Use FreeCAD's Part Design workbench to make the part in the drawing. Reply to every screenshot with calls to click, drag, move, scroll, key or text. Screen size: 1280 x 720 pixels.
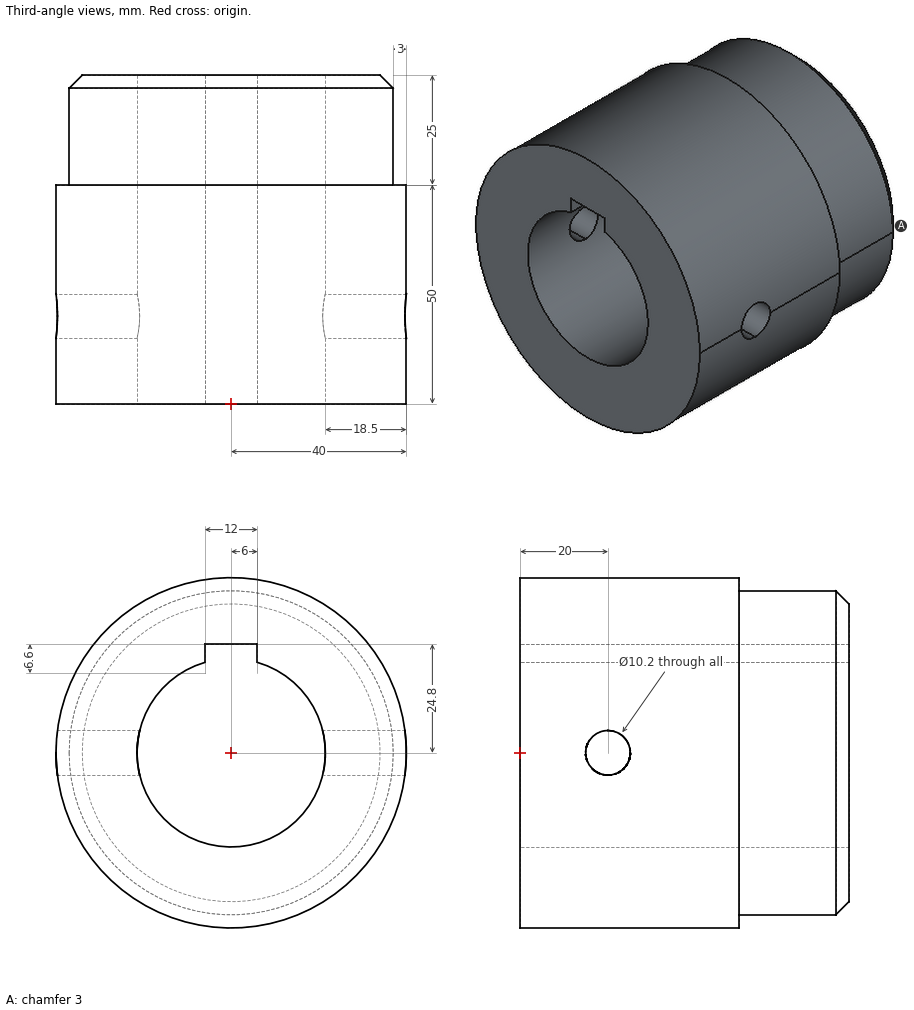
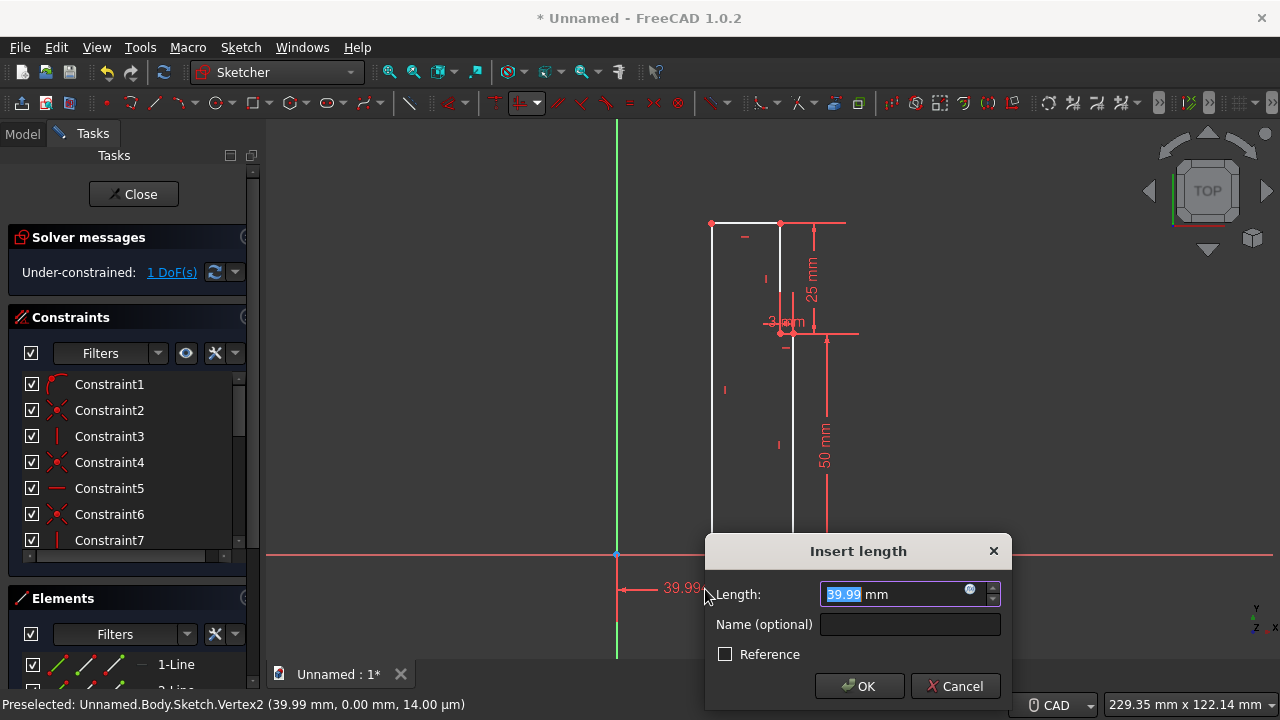
text(40)
key(Return)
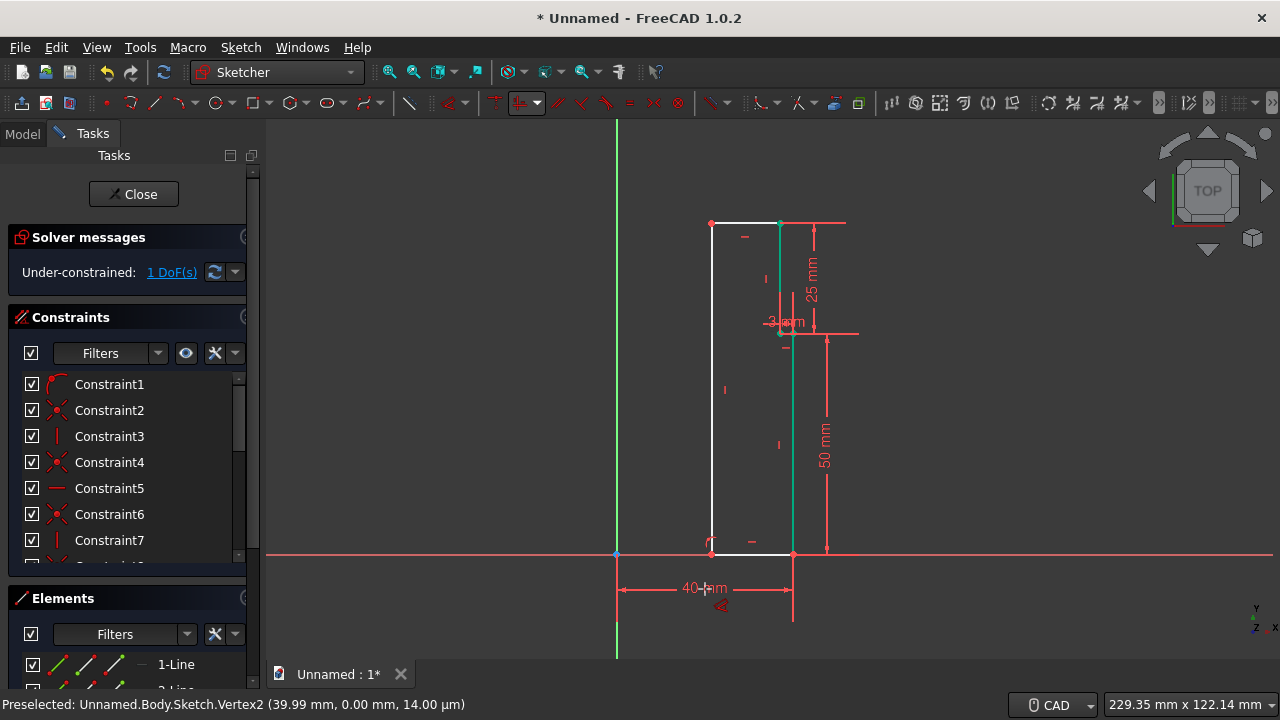
click(736, 555)
click(781, 589)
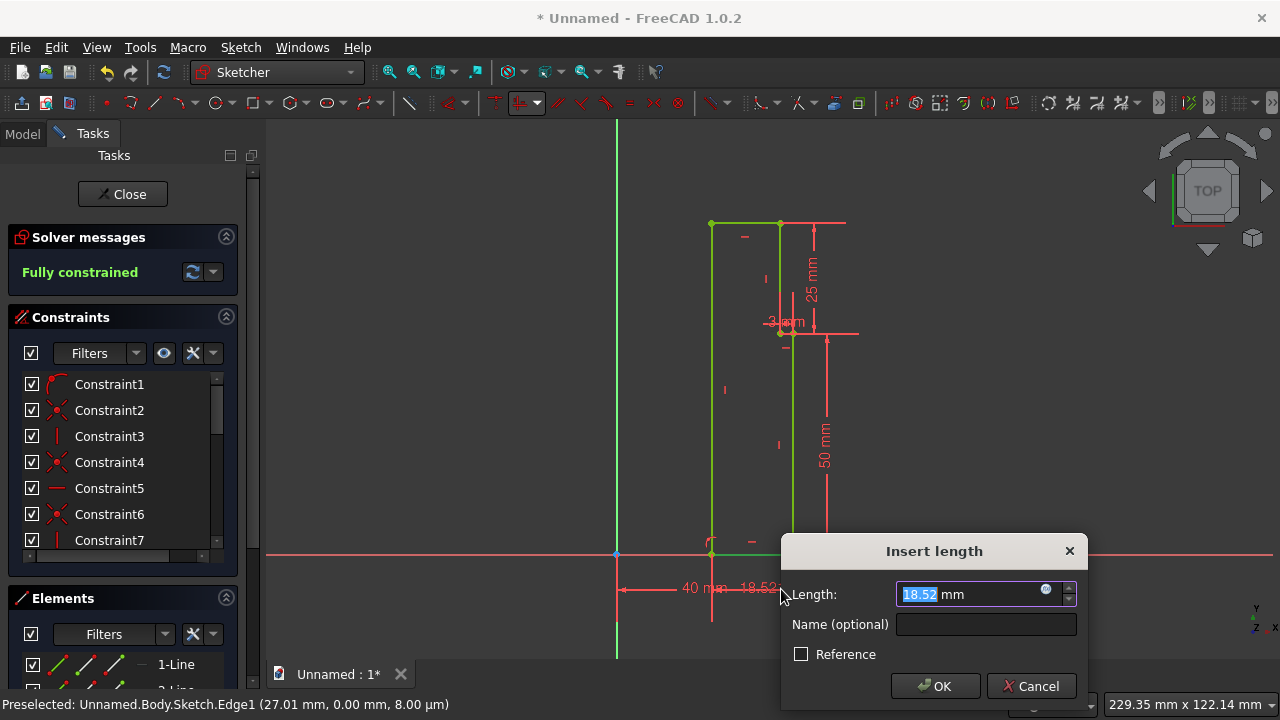
text(18.5)
key(Return)
key(Escape)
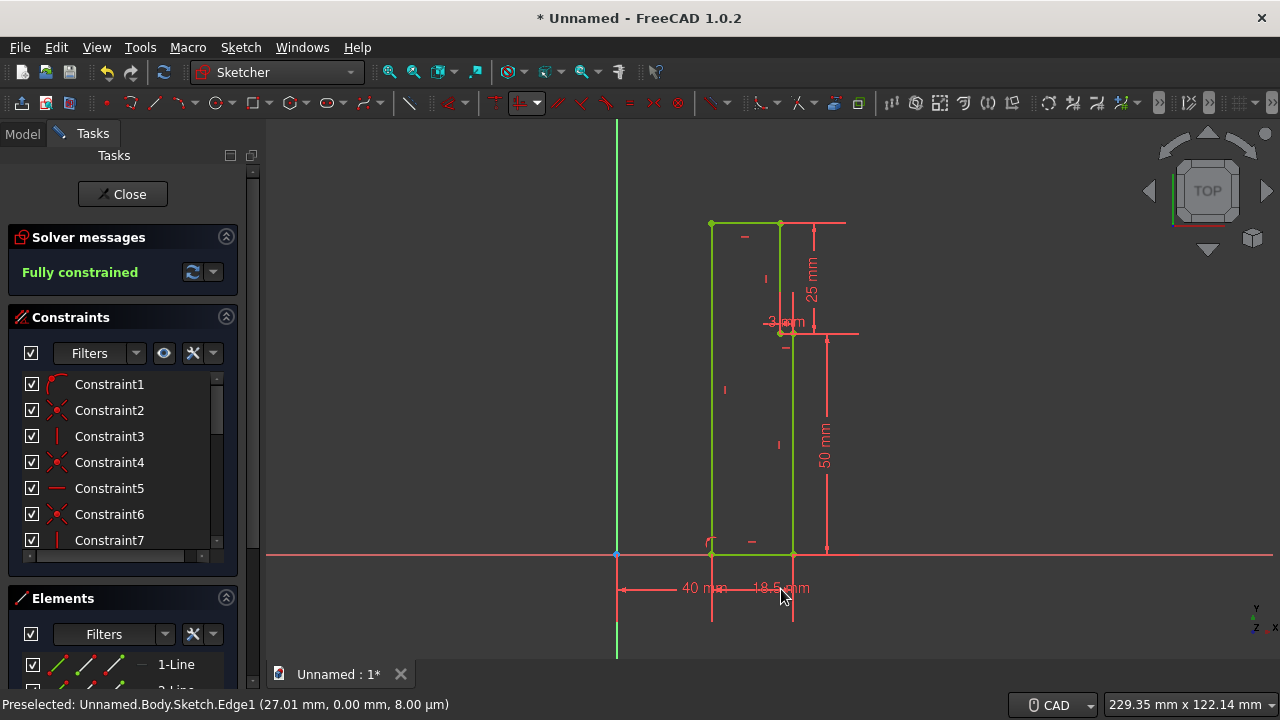
click(123, 194)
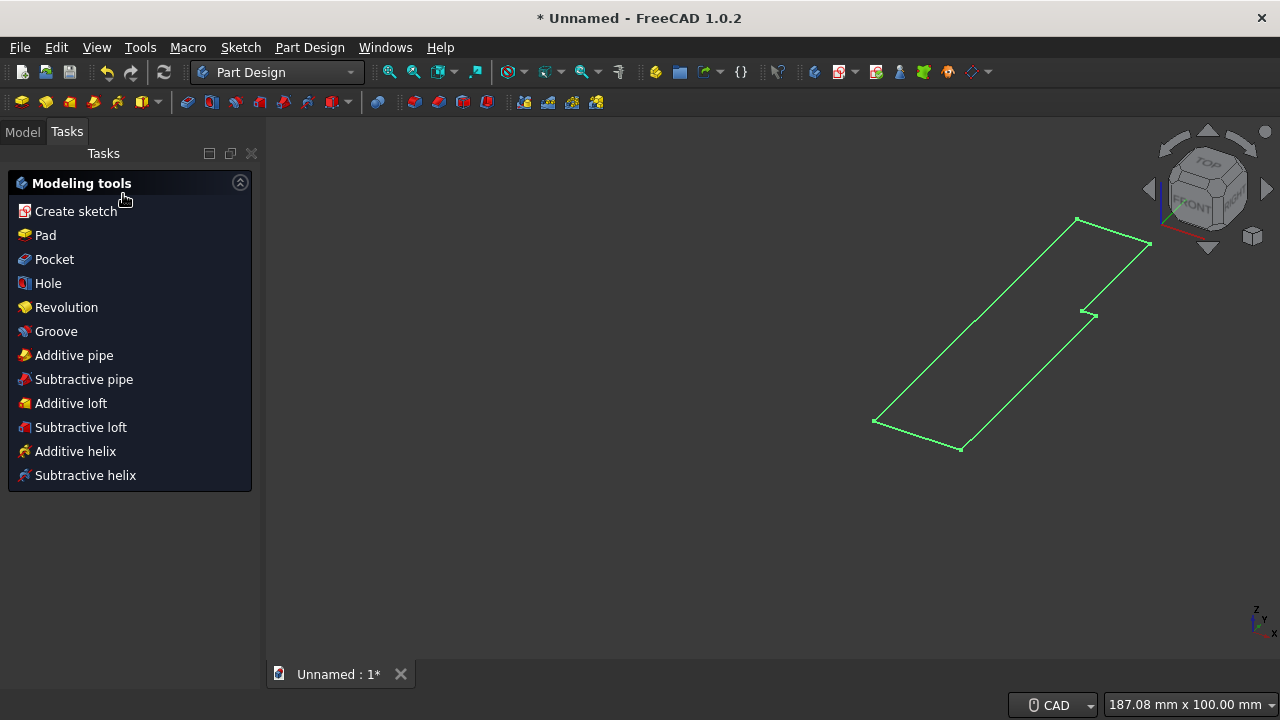
click(46, 102)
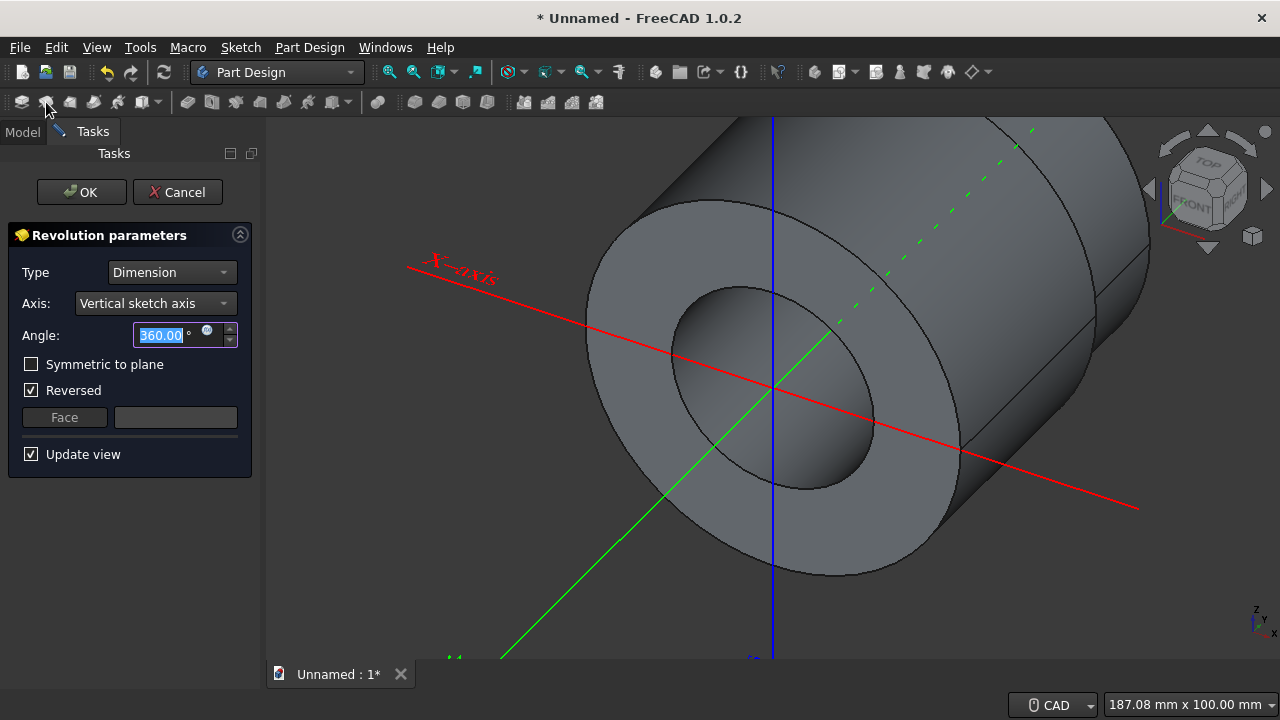
click(82, 192)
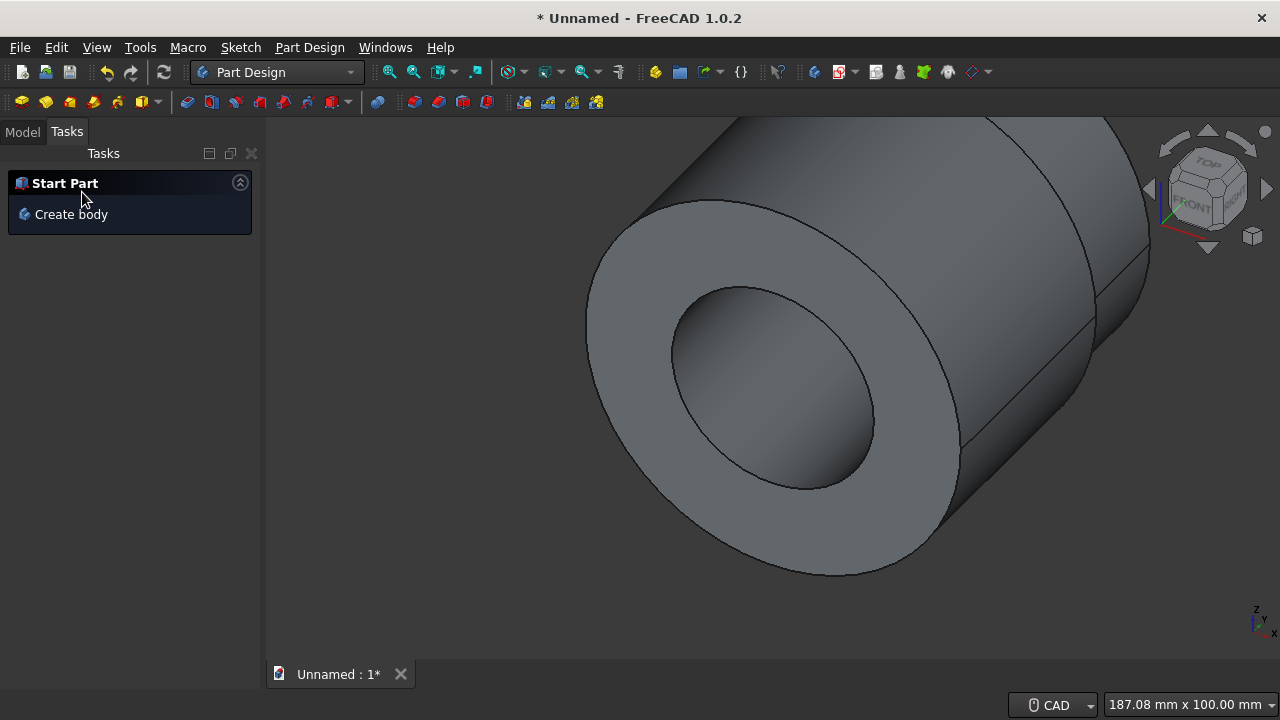
click(390, 72)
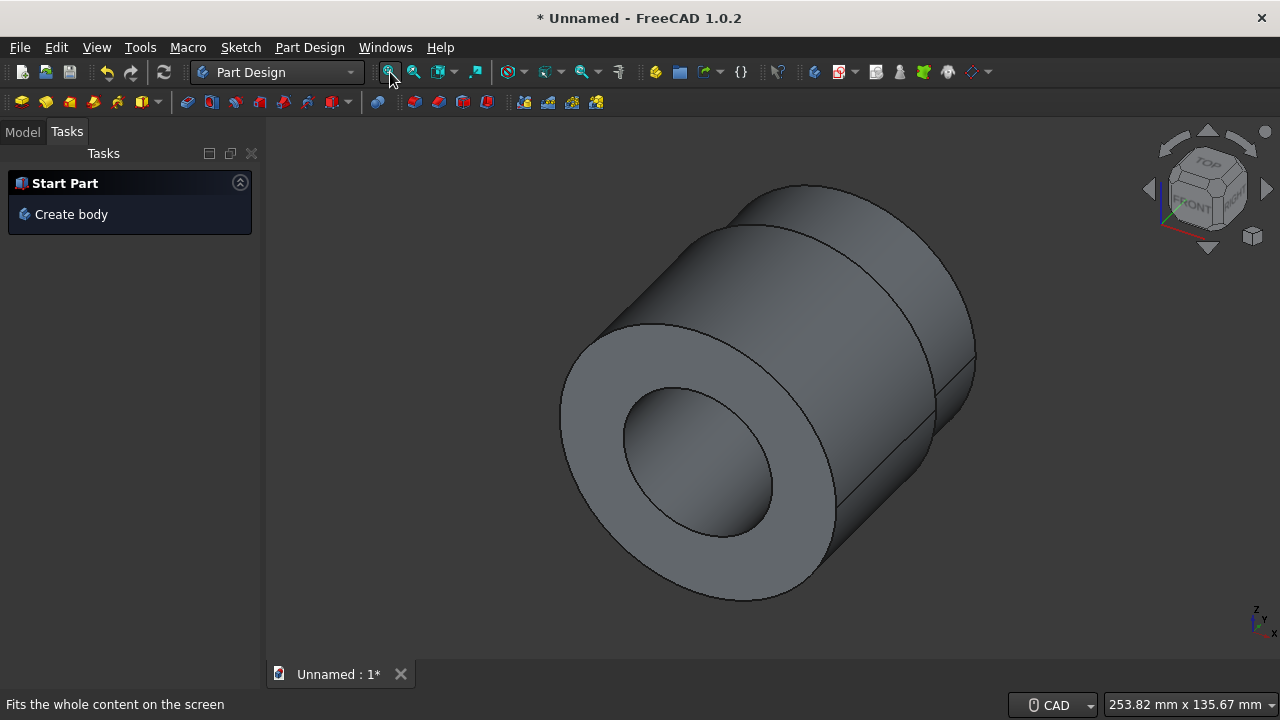
key(0)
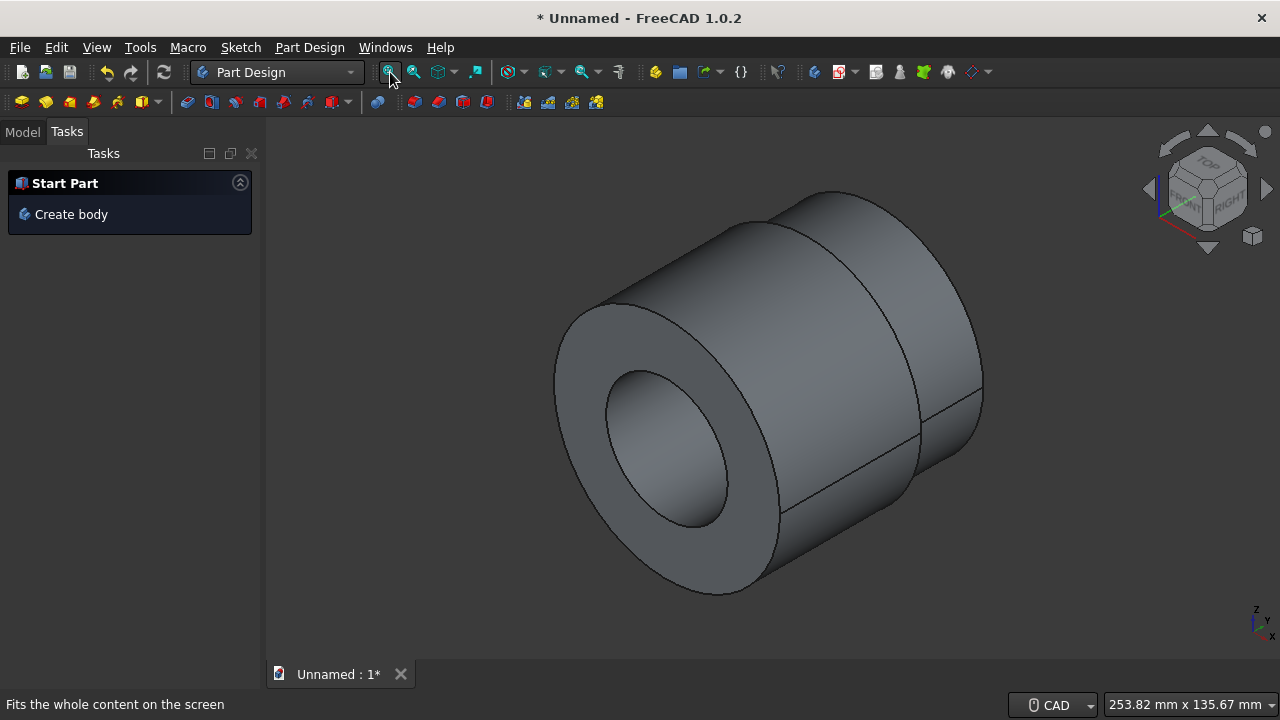
key(2)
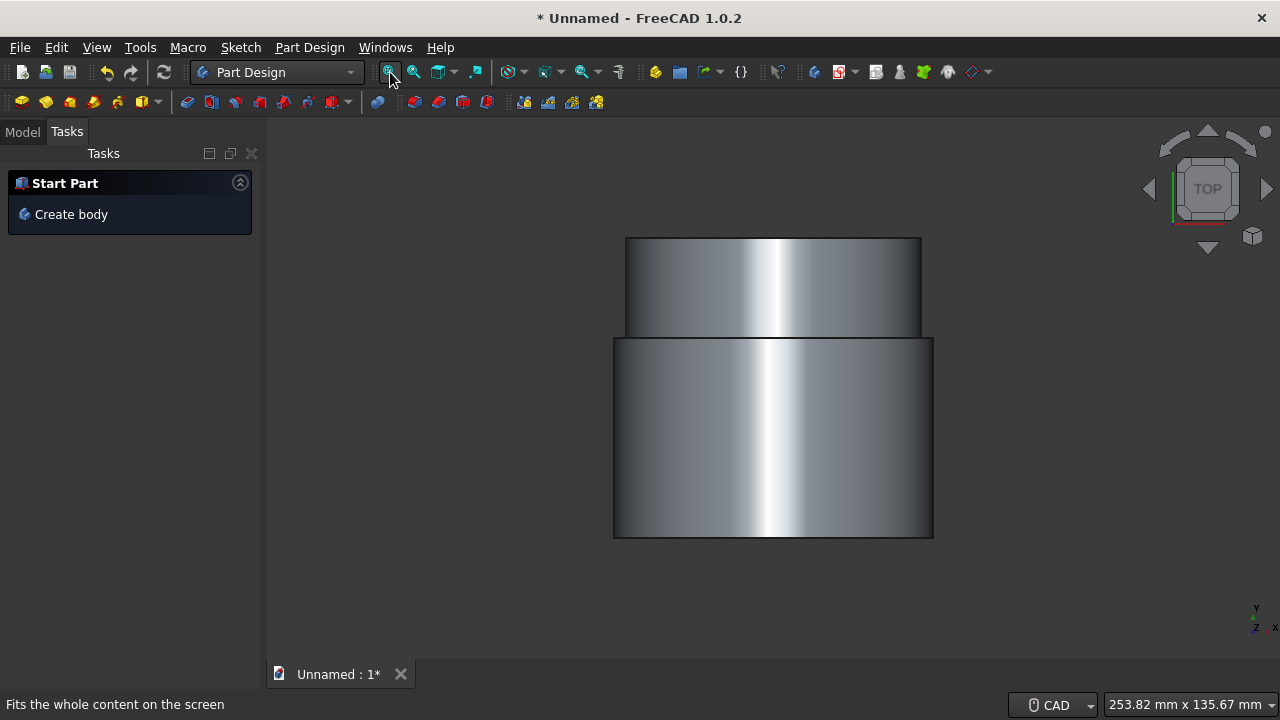
click(653, 237)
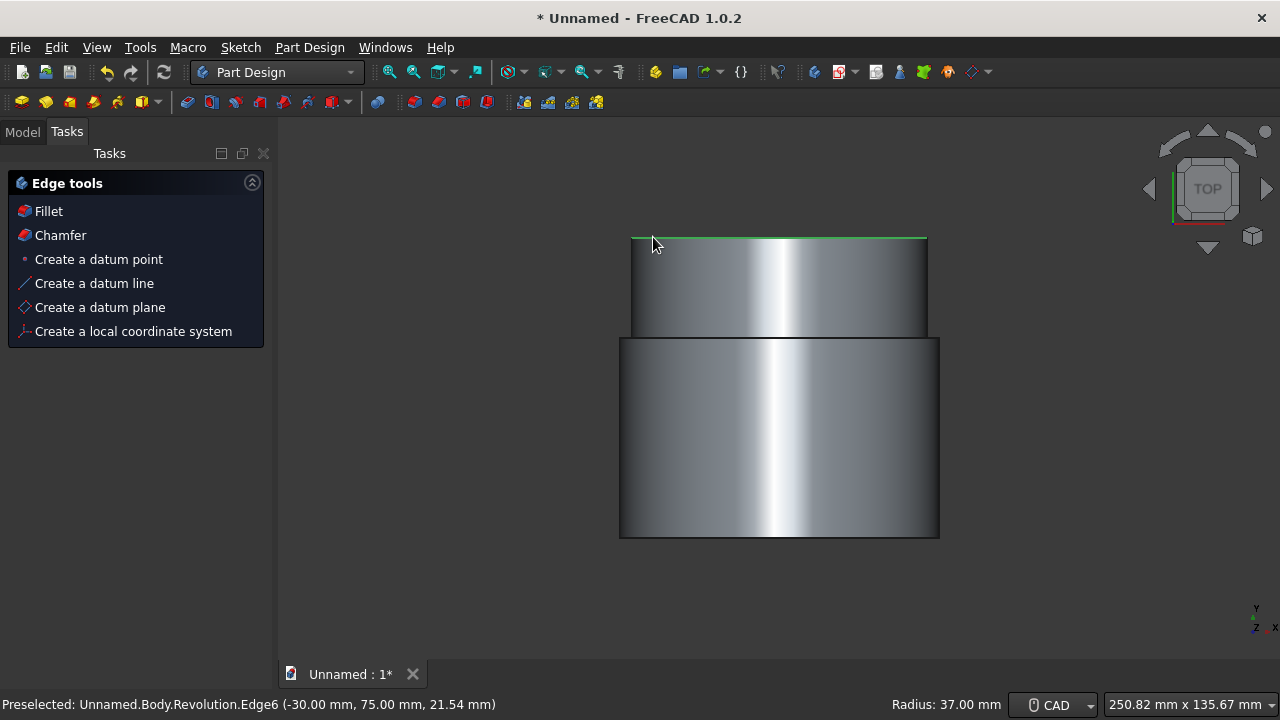
click(440, 102)